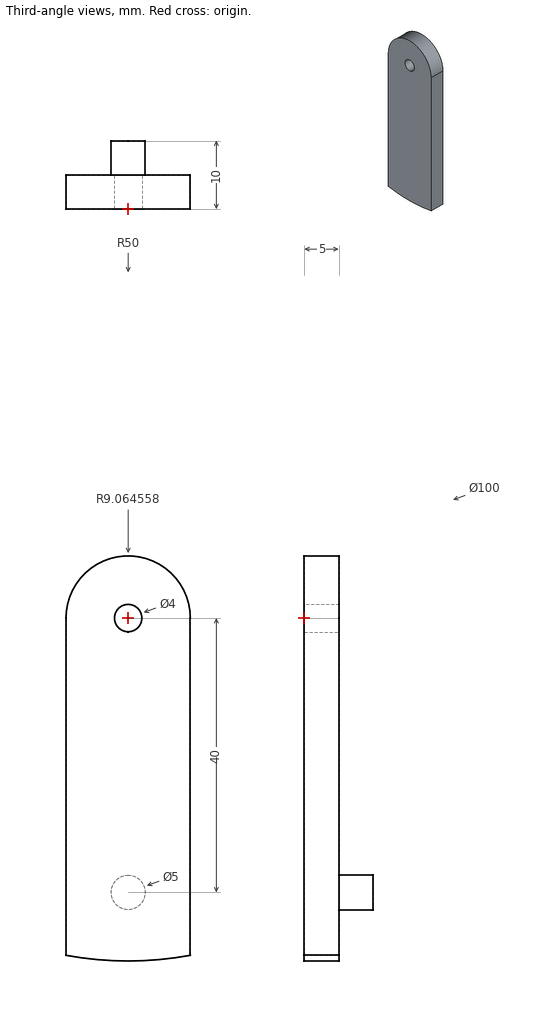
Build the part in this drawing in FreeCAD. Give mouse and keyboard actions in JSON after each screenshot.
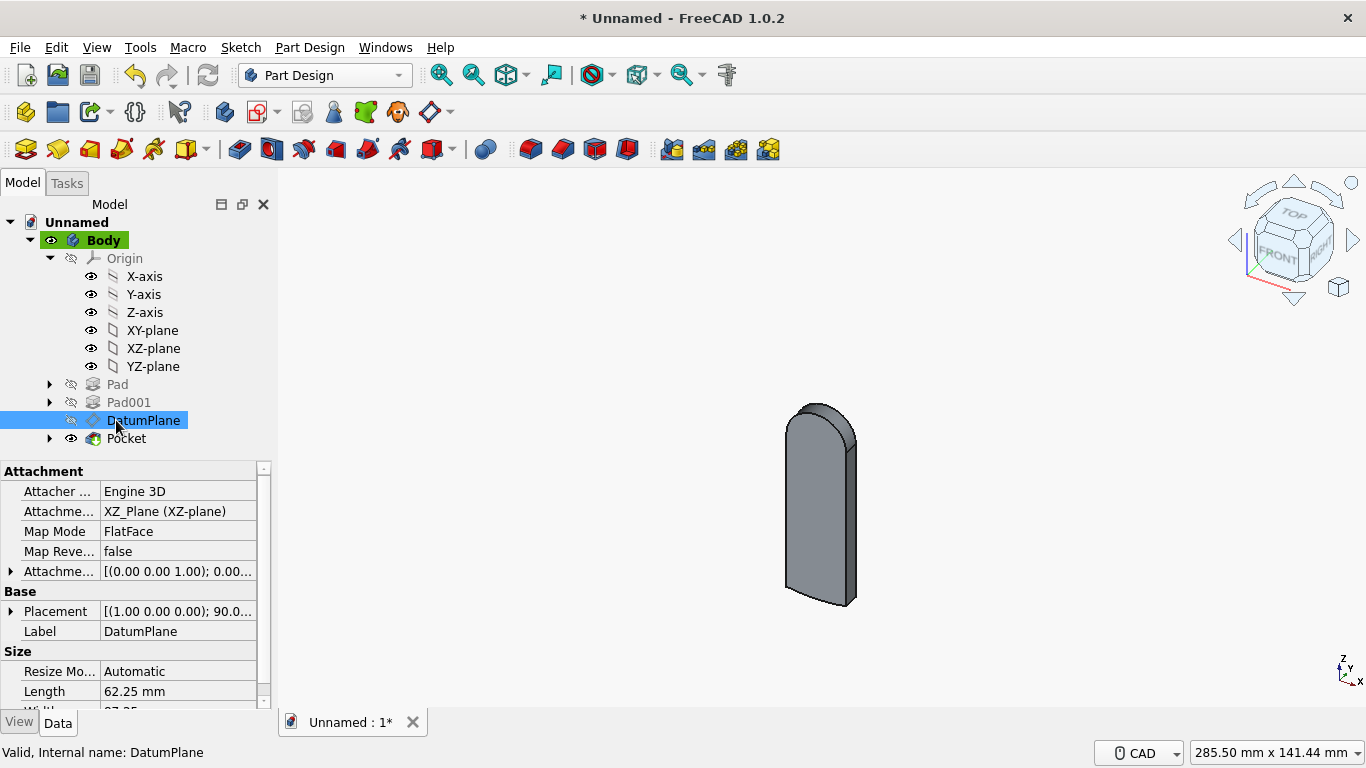
{"action": "key", "text": "v f"}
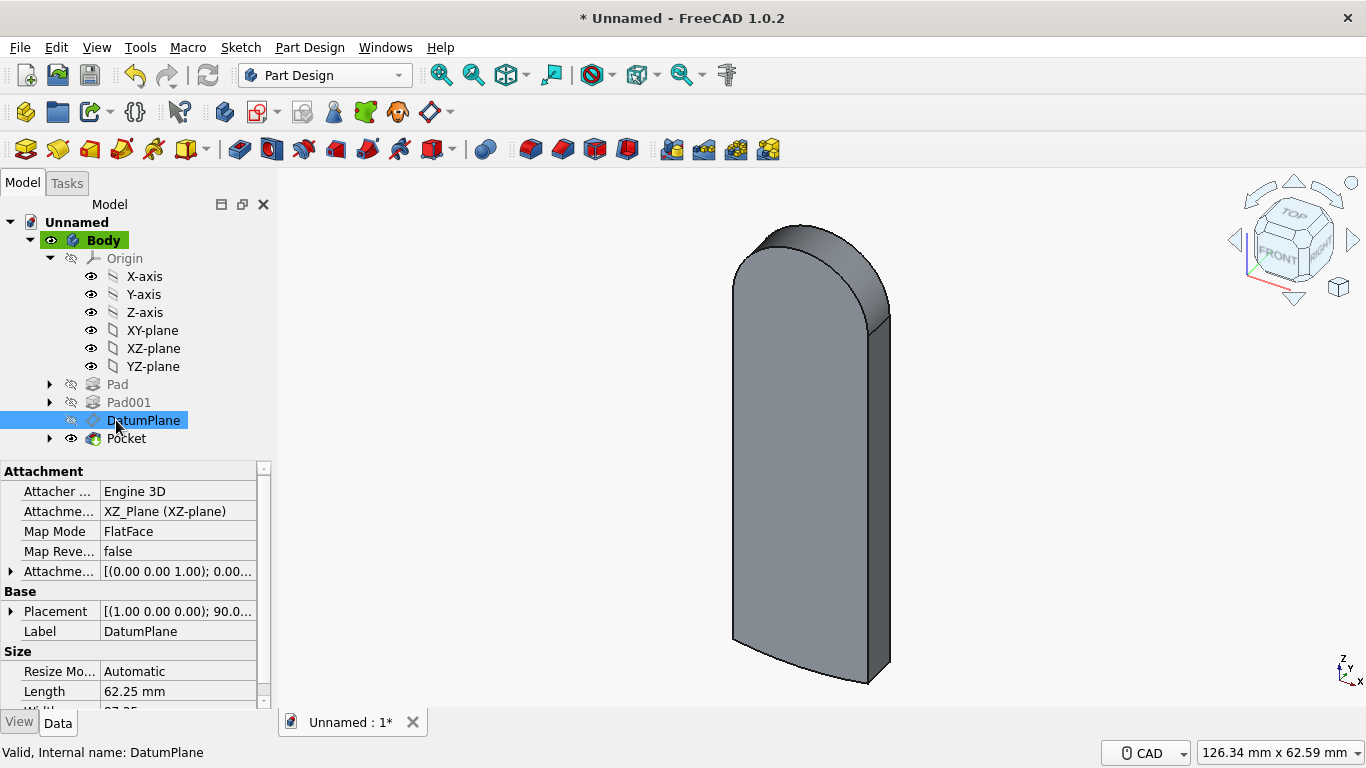
{"action": "left_click", "coordinate": [800, 339]}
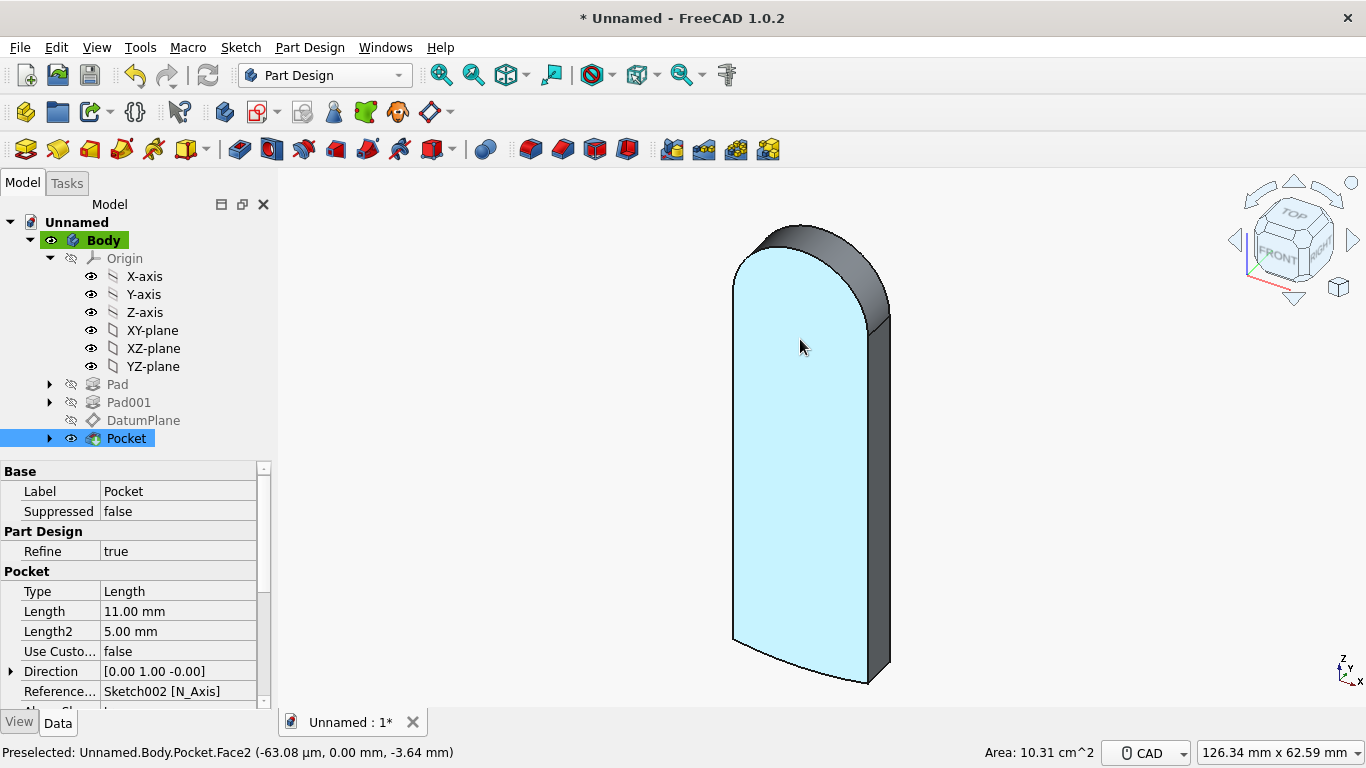
{"action": "left_click", "coordinate": [258, 112]}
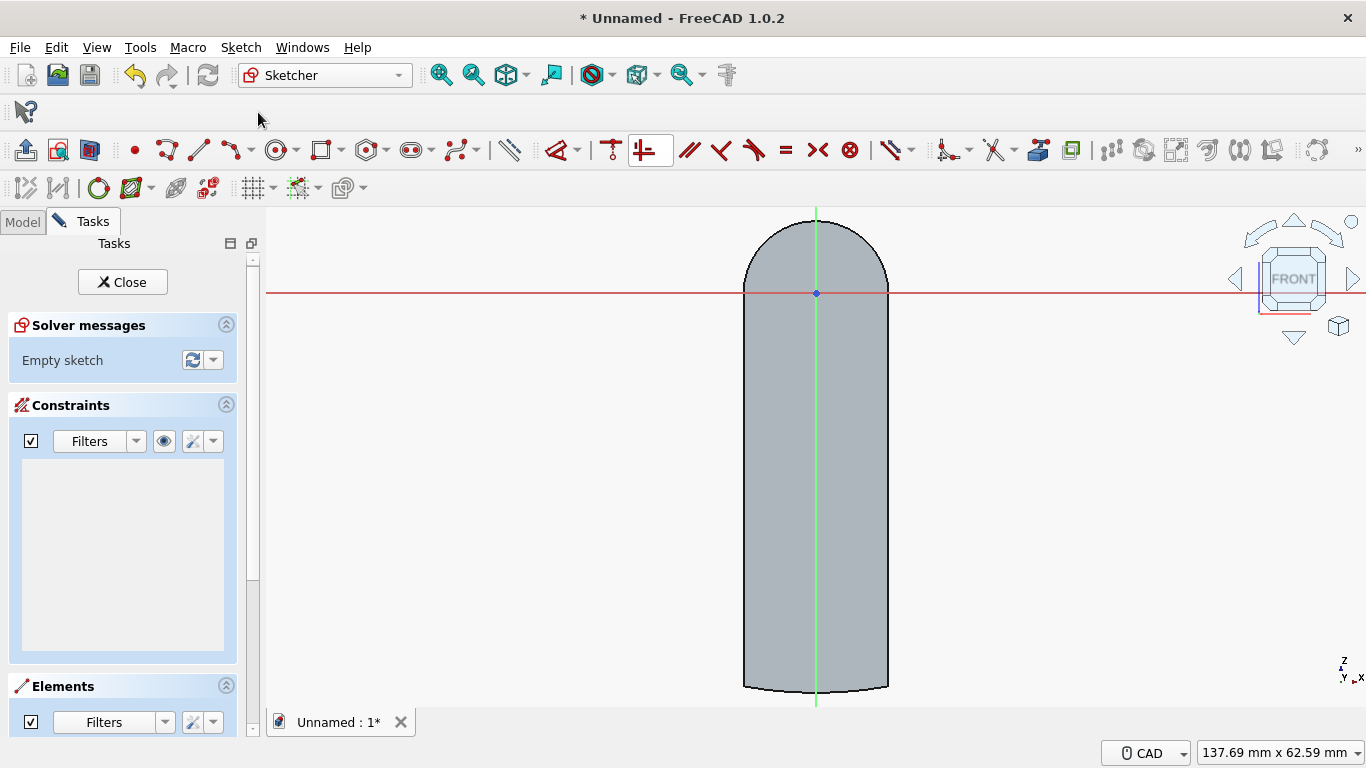
{"action": "scroll", "coordinate": [825, 273], "scroll_direction": "up", "scroll_amount": 11}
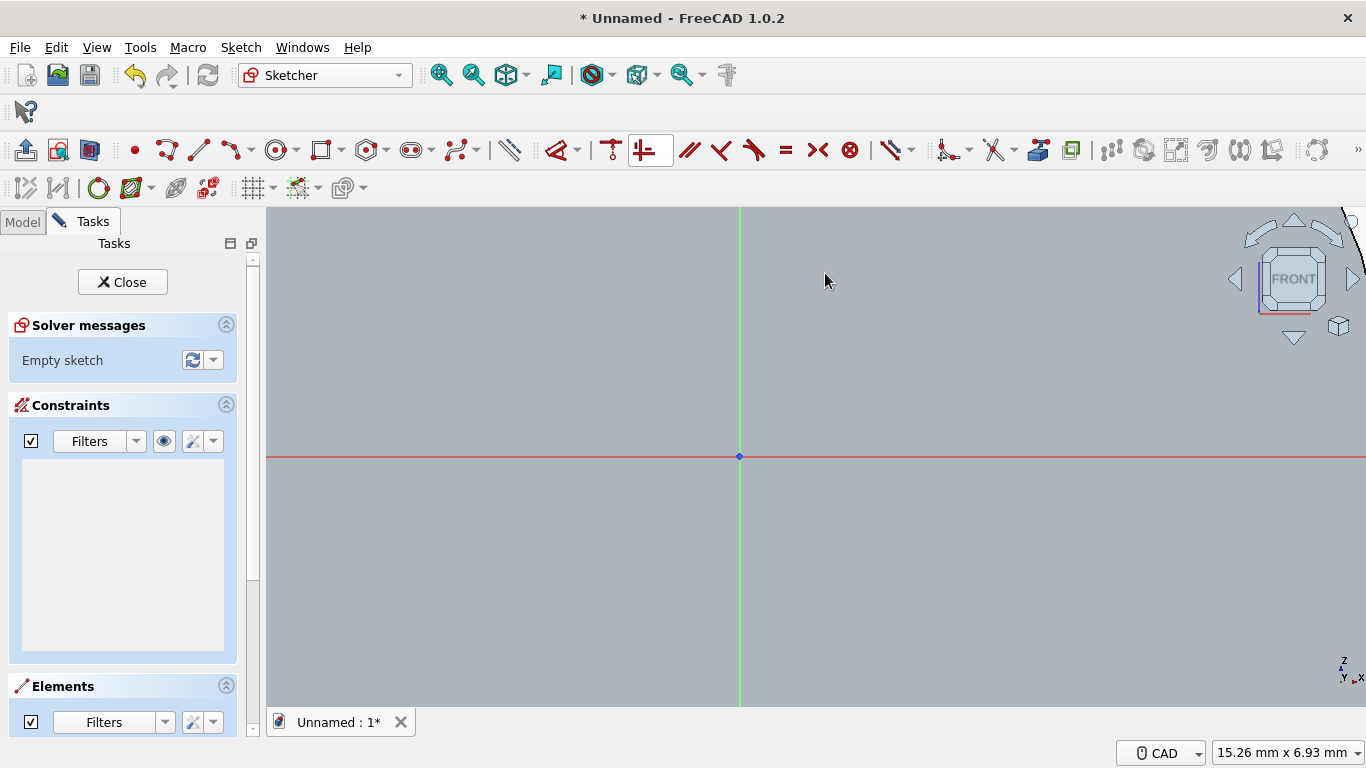
{"action": "left_click", "coordinate": [276, 150]}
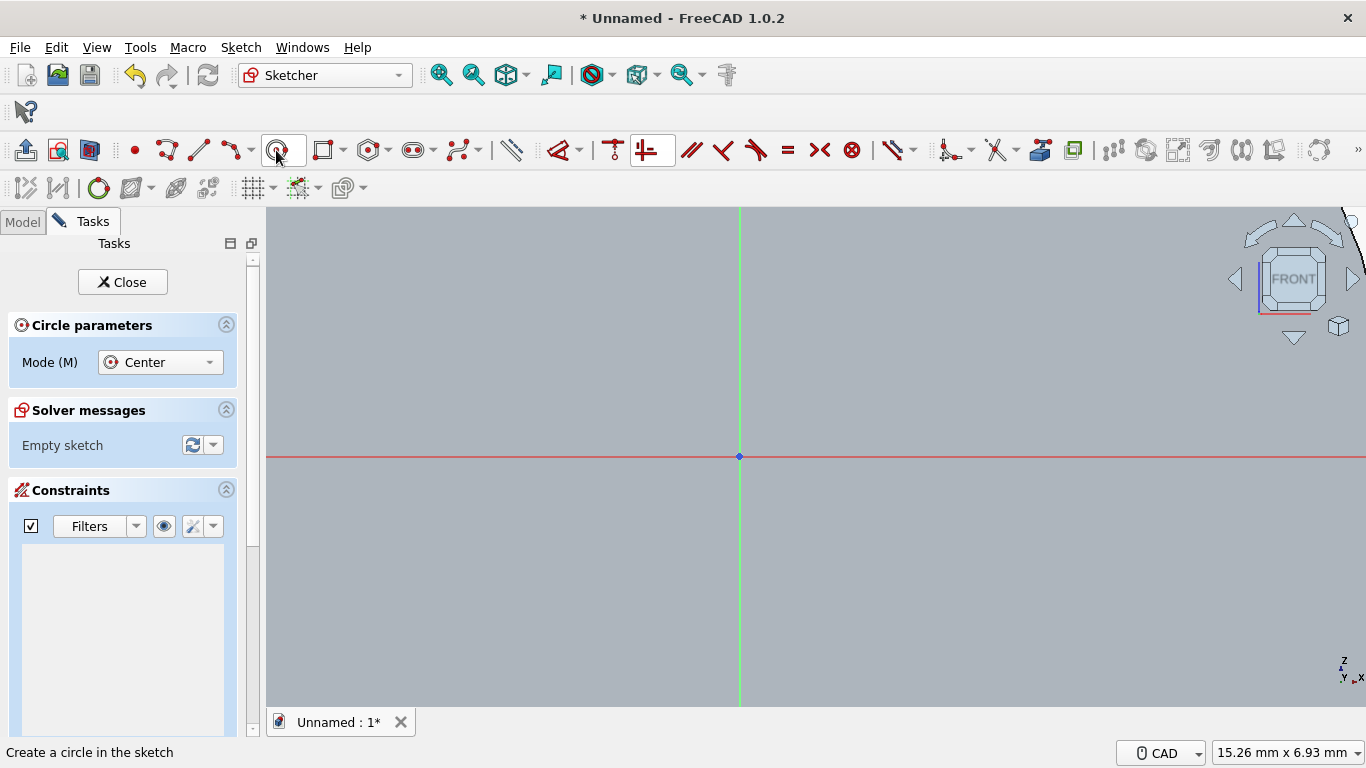
{"action": "left_click", "coordinate": [740, 457]}
{"action": "left_click", "coordinate": [842, 355]}
{"action": "key", "text": "Escape"}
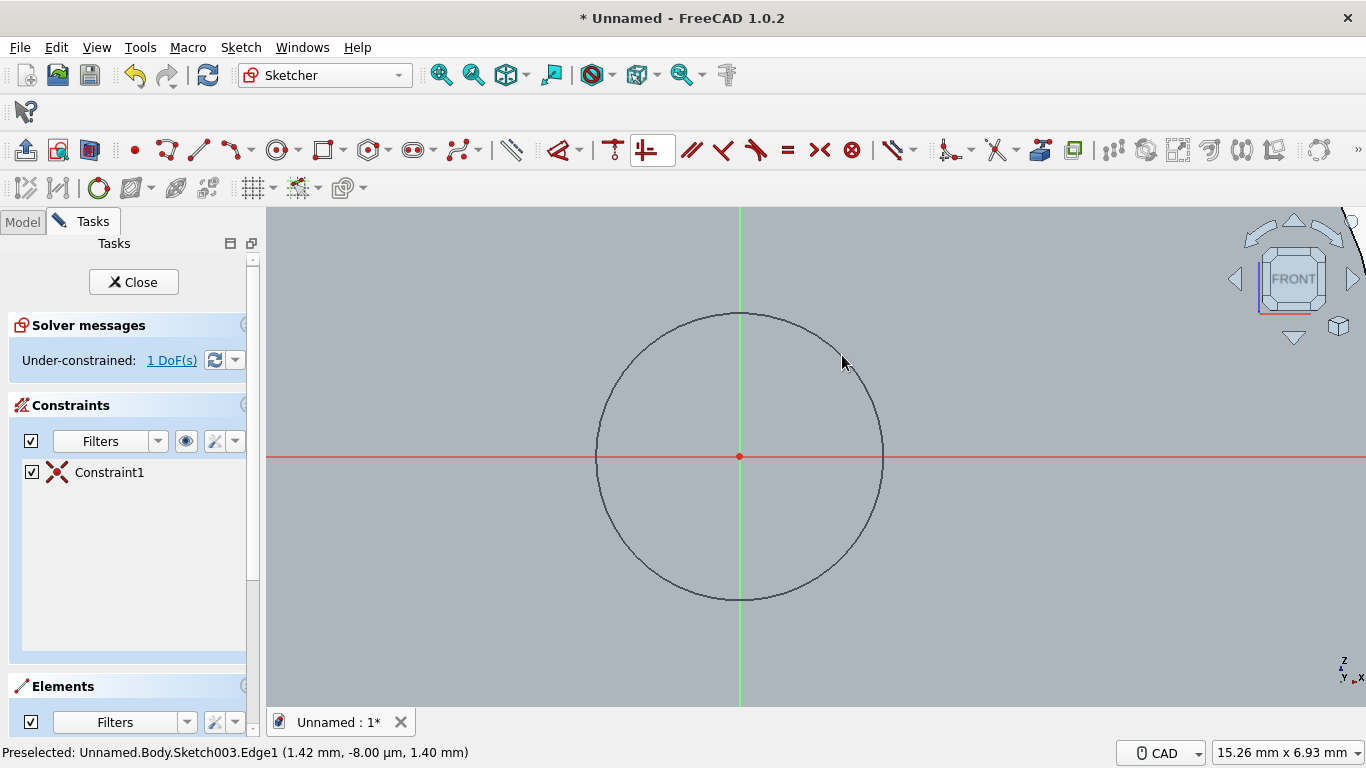
{"action": "left_click", "coordinate": [841, 355]}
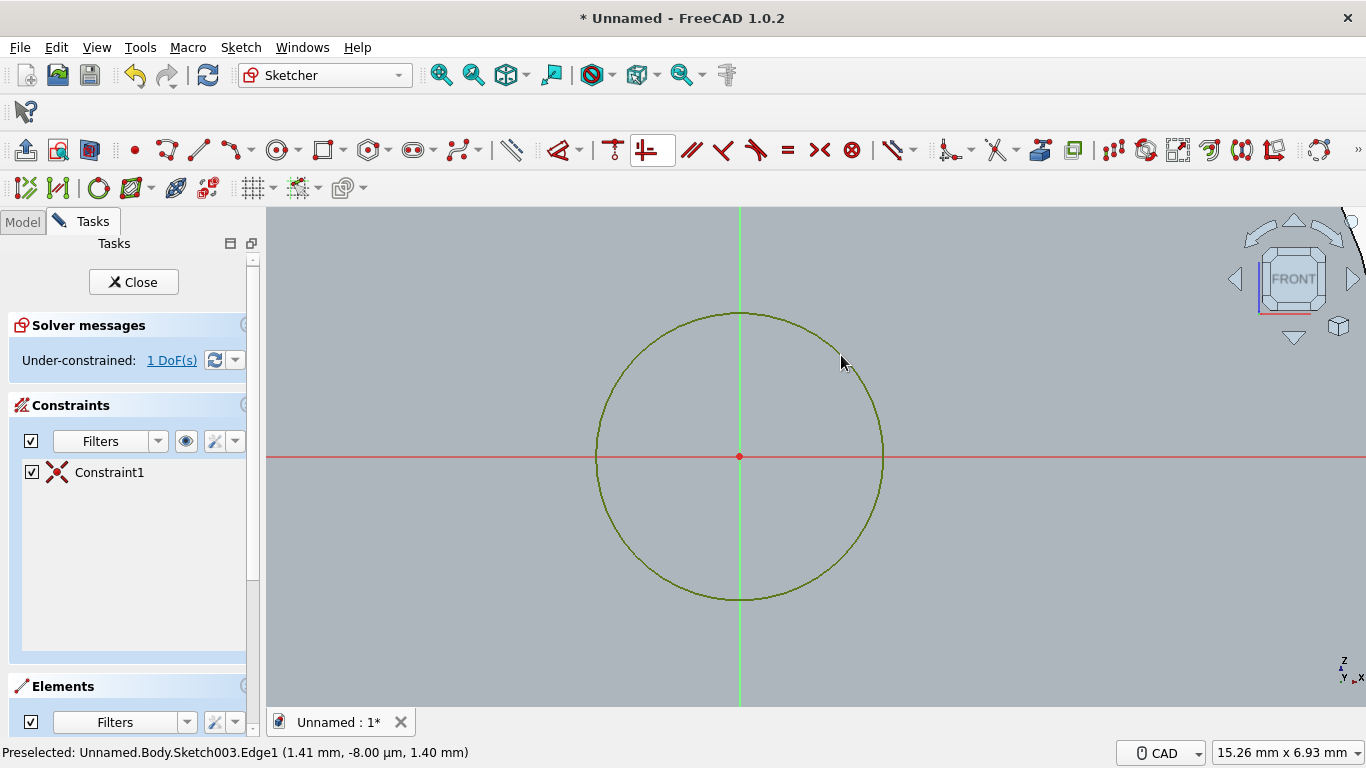
{"action": "key", "text": "k o"}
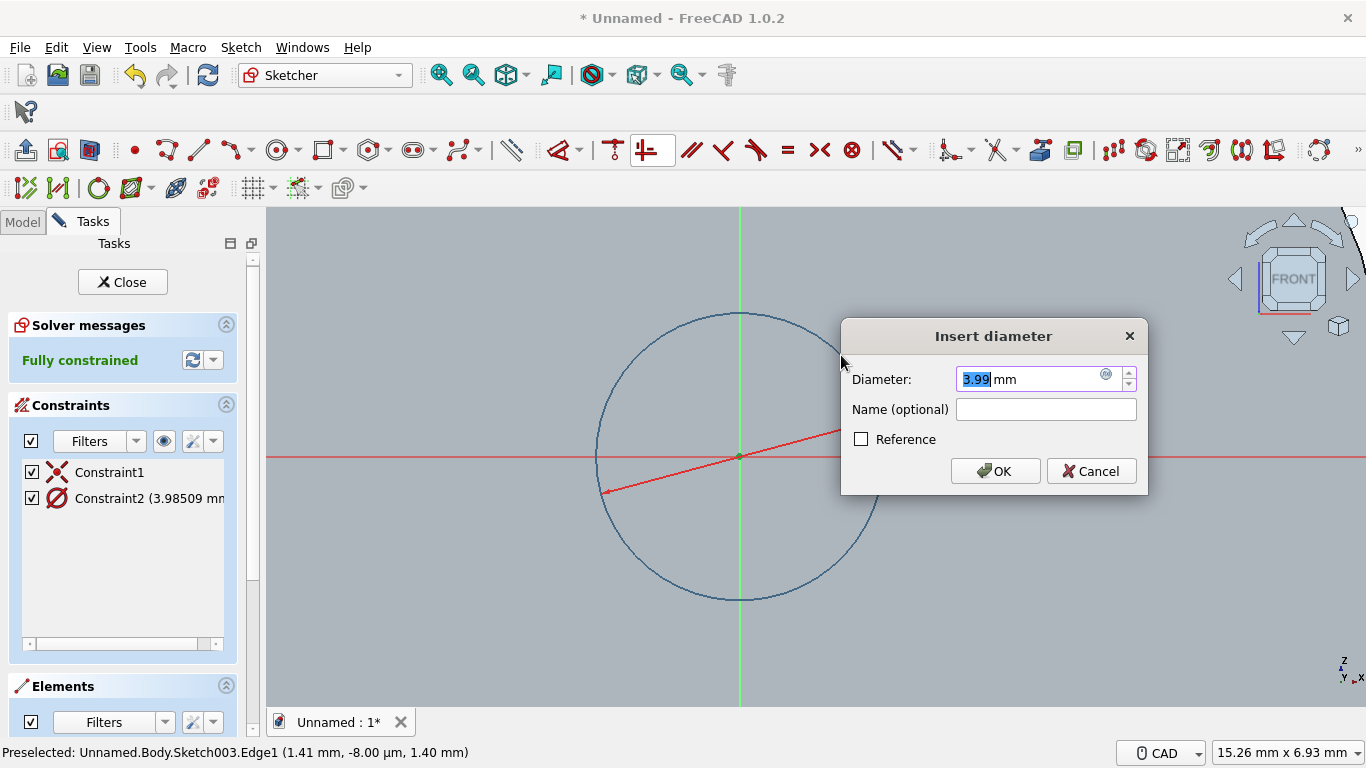
{"action": "type", "text": "4"}
{"action": "key", "text": "Return"}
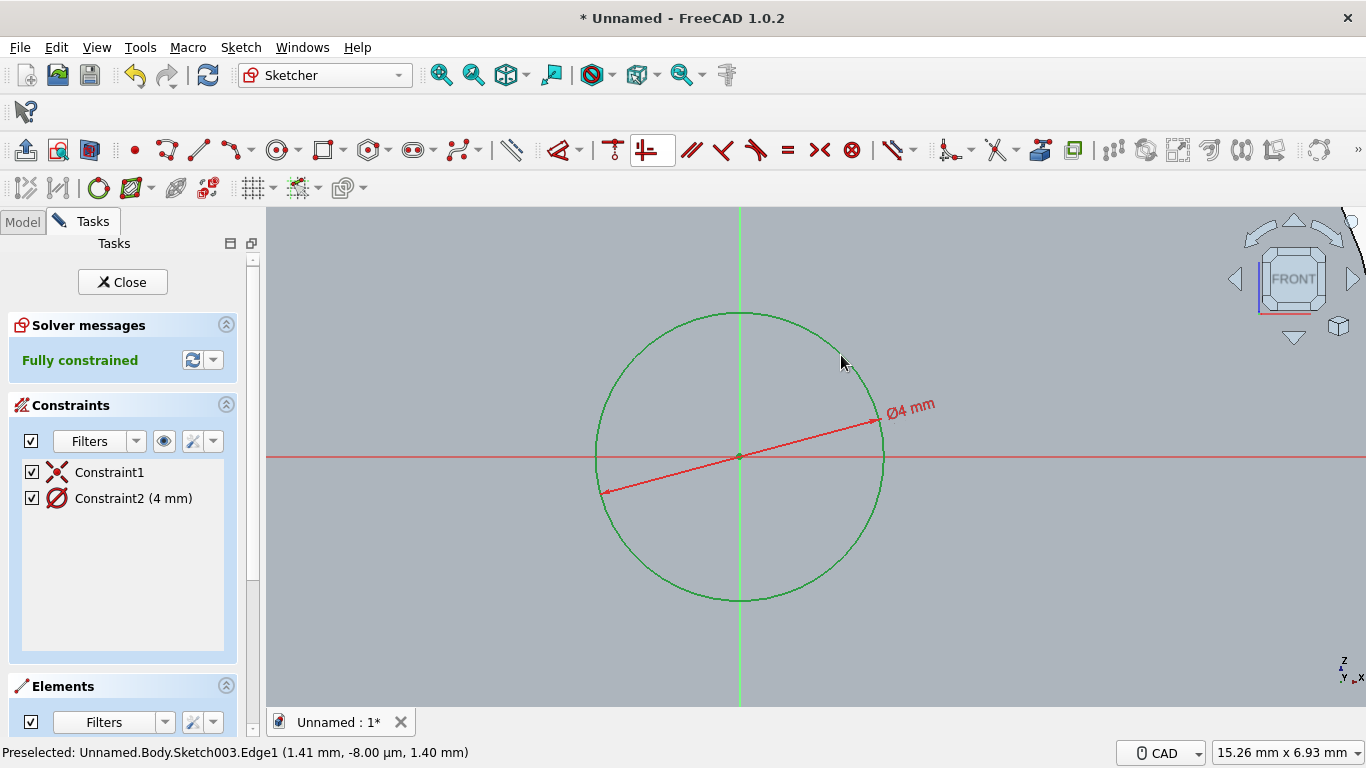
{"action": "left_click", "coordinate": [123, 282]}